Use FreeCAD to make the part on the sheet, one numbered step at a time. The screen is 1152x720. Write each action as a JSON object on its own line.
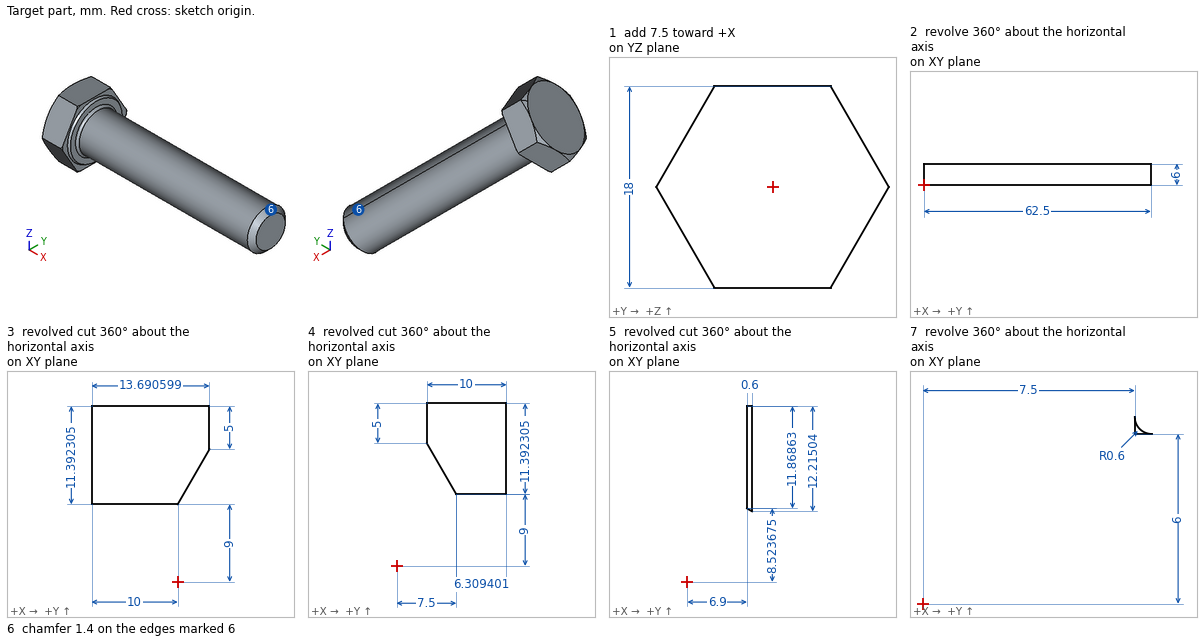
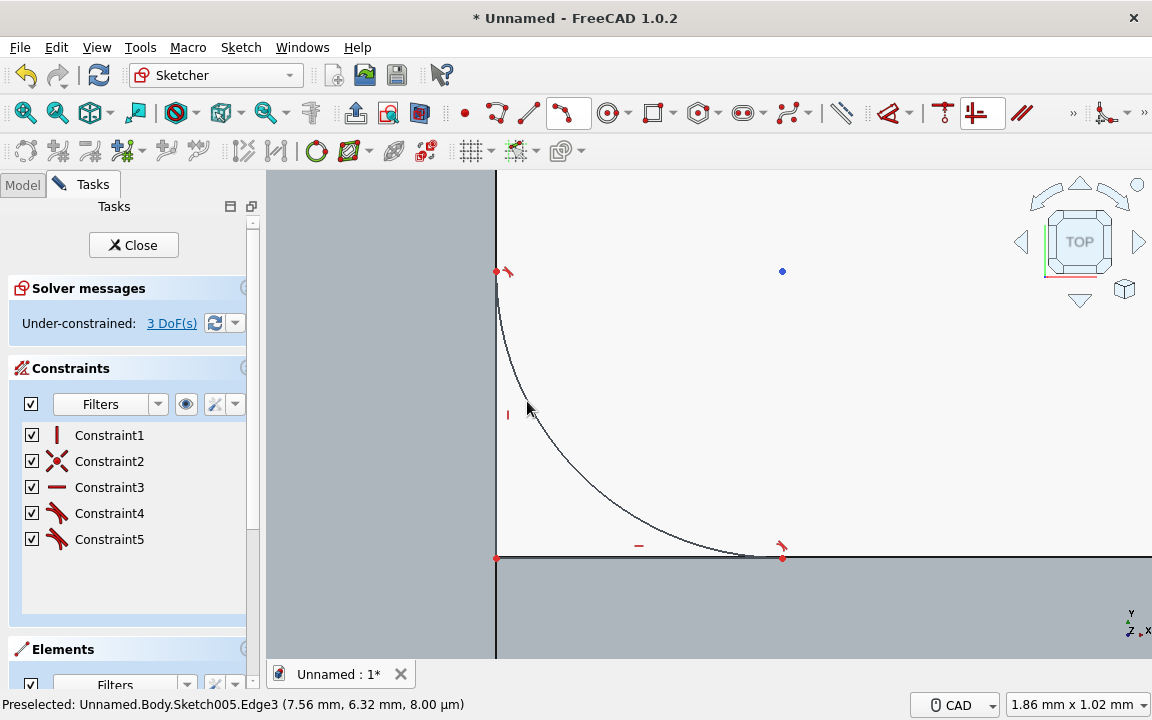
{"action": "key", "text": "d"}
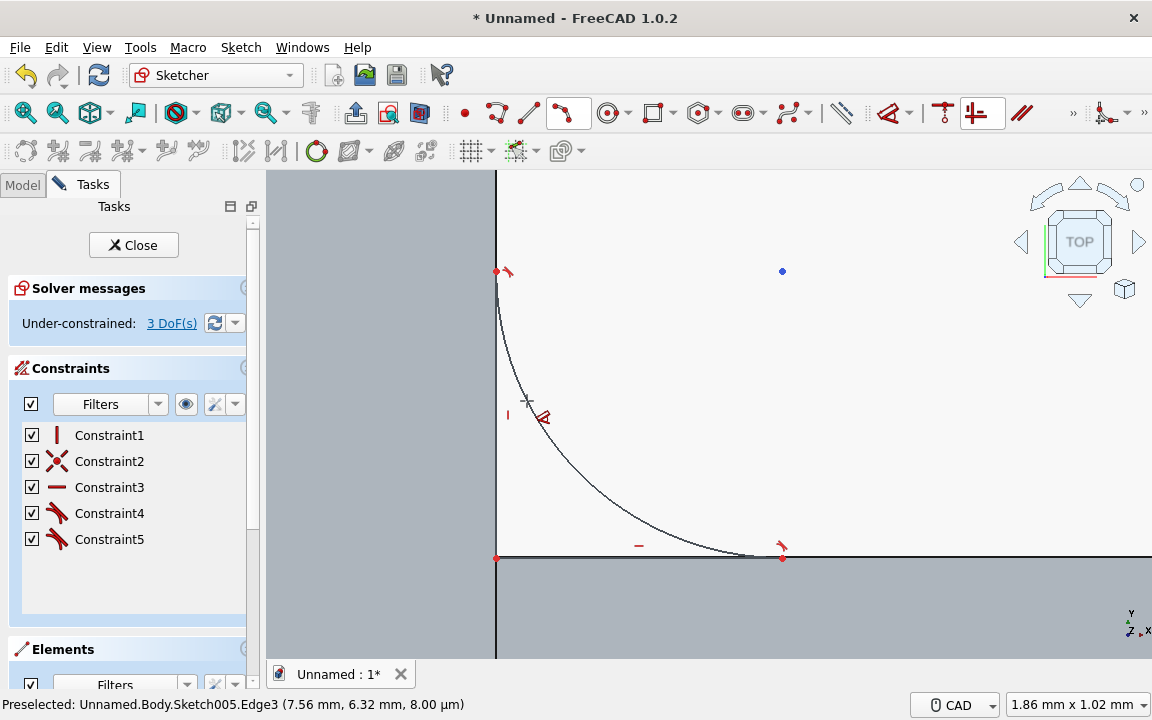
{"action": "left_click", "coordinate": [527, 401]}
{"action": "left_click", "coordinate": [464, 261]}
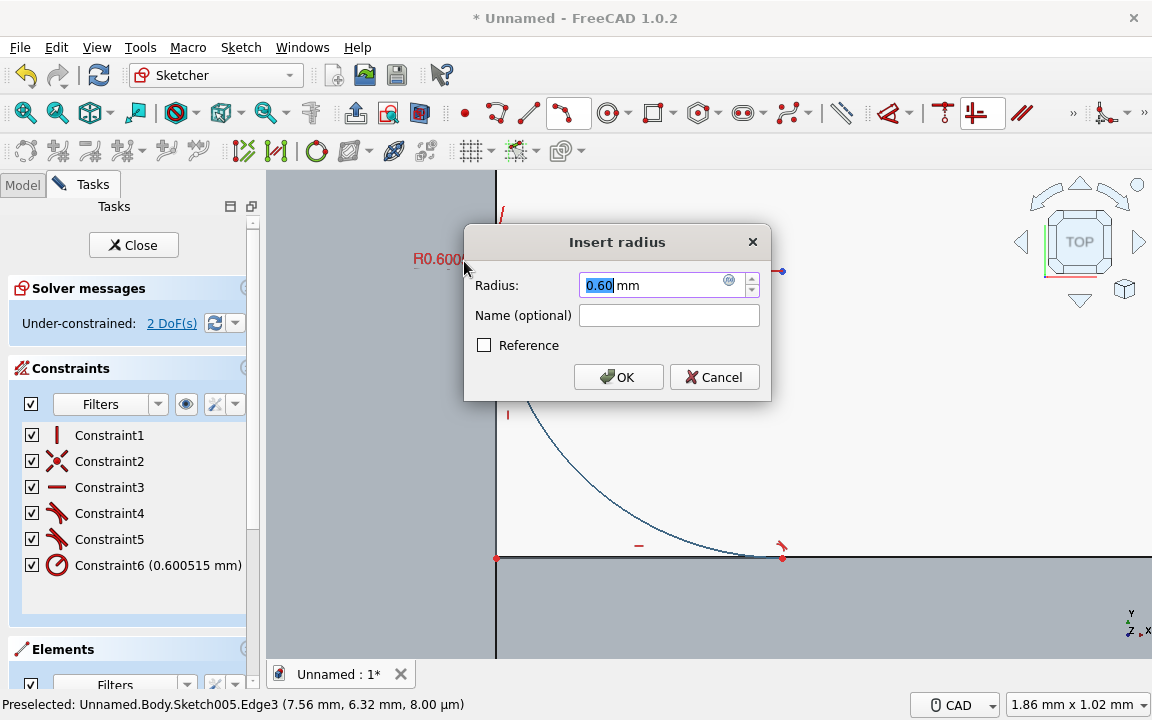
{"action": "type", "text": "0.6"}
{"action": "key", "text": "Return"}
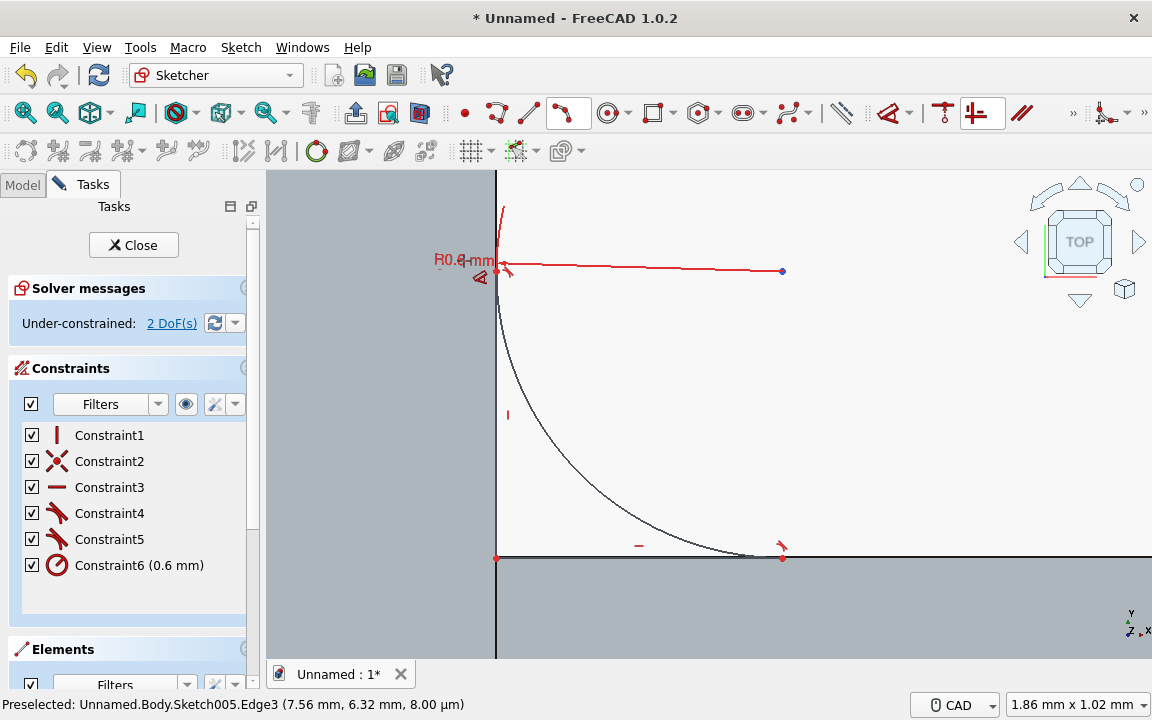
{"action": "left_click", "coordinate": [496, 558]}
{"action": "left_click", "coordinate": [530, 595]}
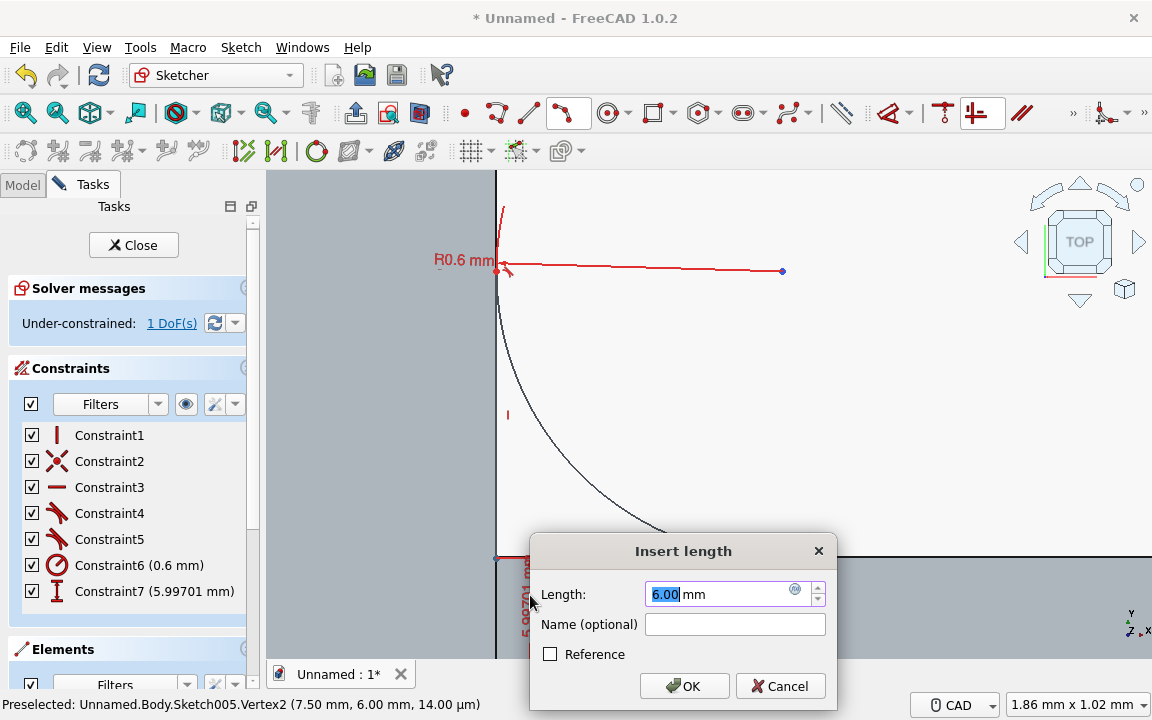
{"action": "type", "text": "6"}
{"action": "key", "text": "Return"}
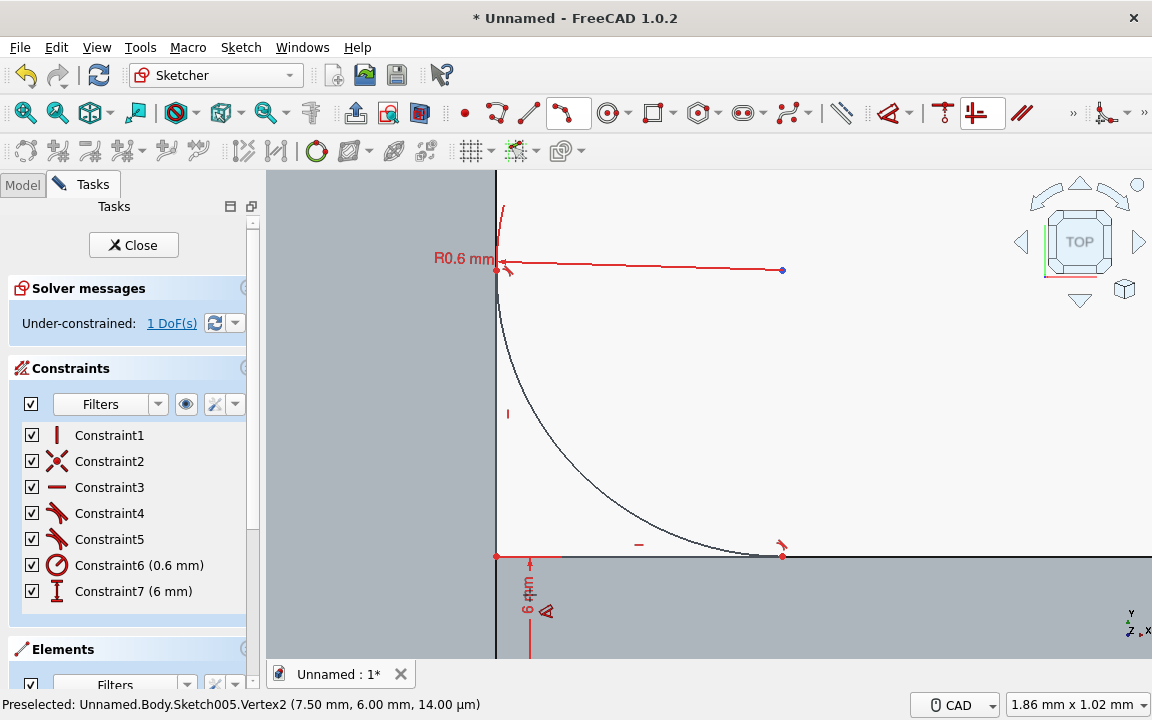
{"action": "left_click", "coordinate": [496, 270]}
{"action": "left_click", "coordinate": [395, 236]}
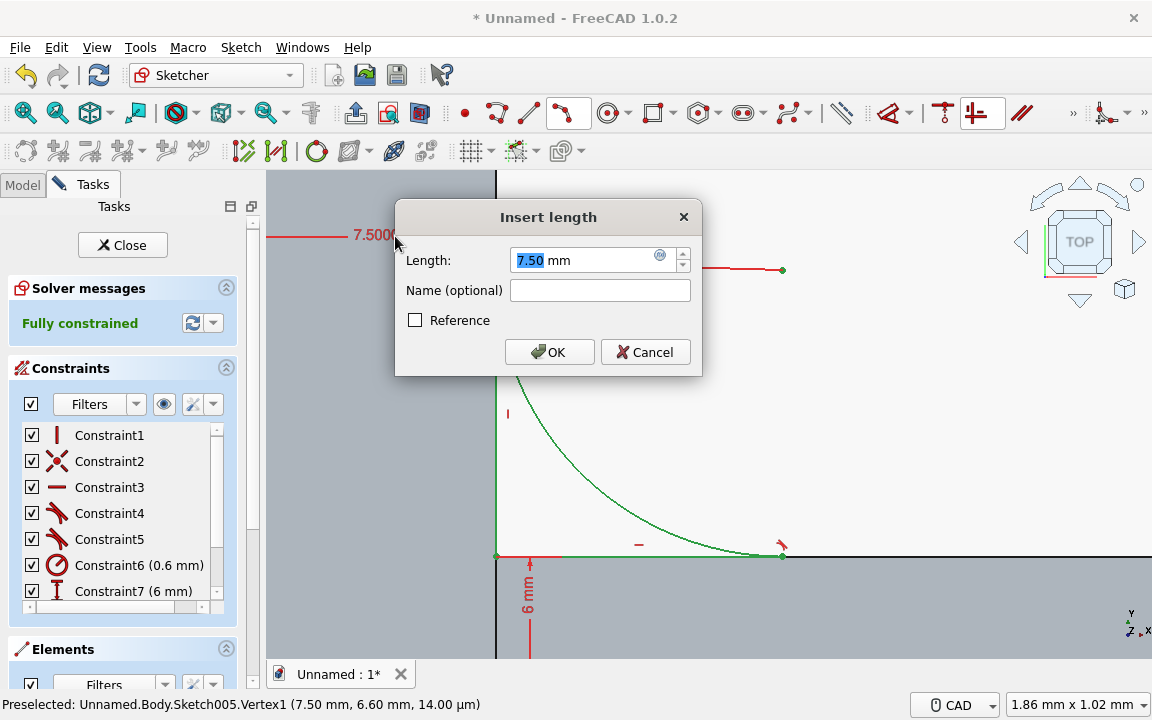
{"action": "type", "text": "7.5"}
{"action": "key", "text": "Return"}
{"action": "key", "text": "Escape"}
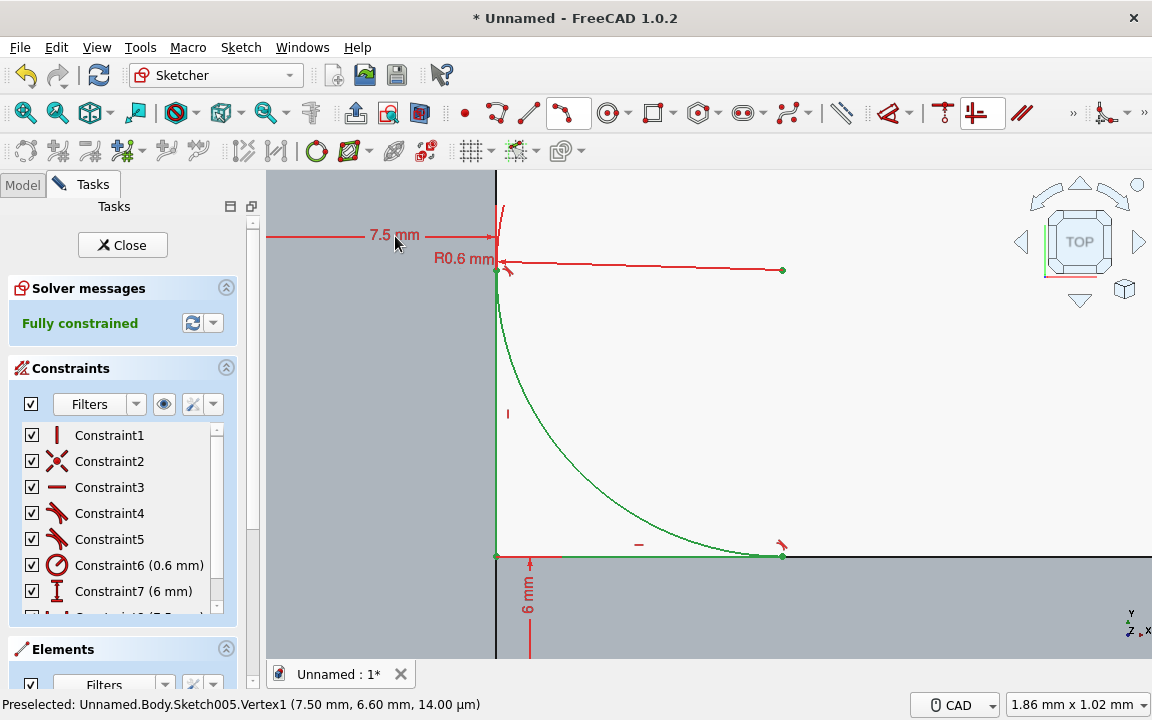
{"action": "left_click", "coordinate": [123, 245]}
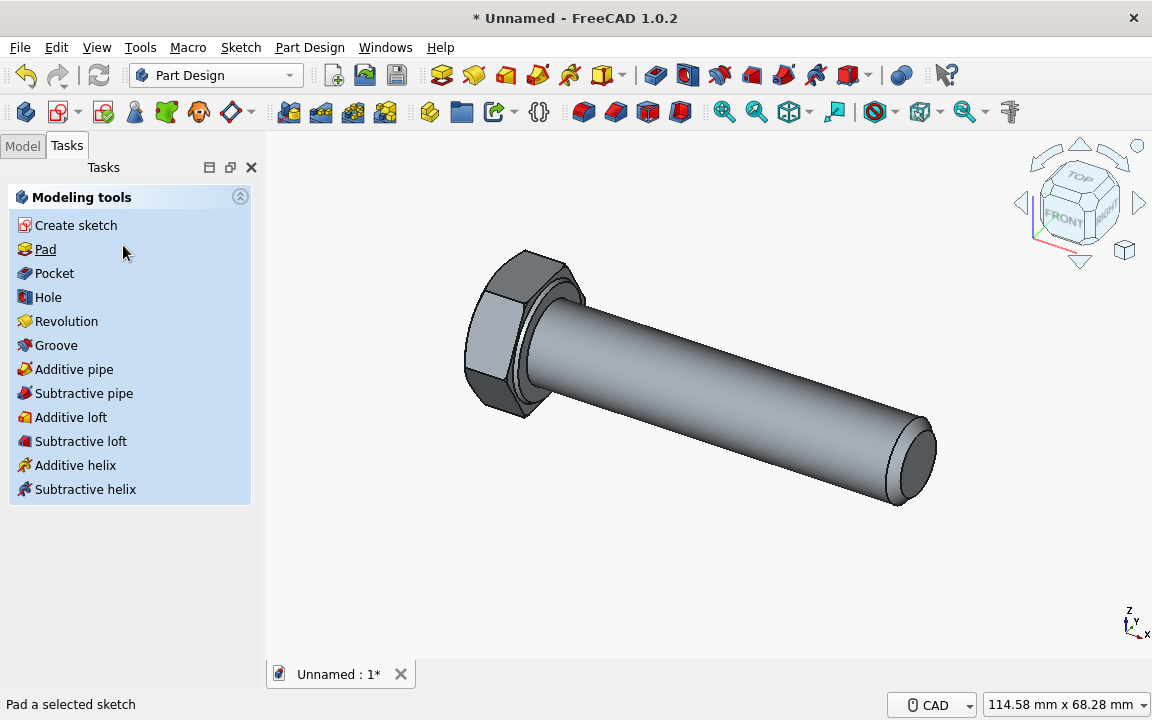
{"action": "left_click", "coordinate": [474, 76]}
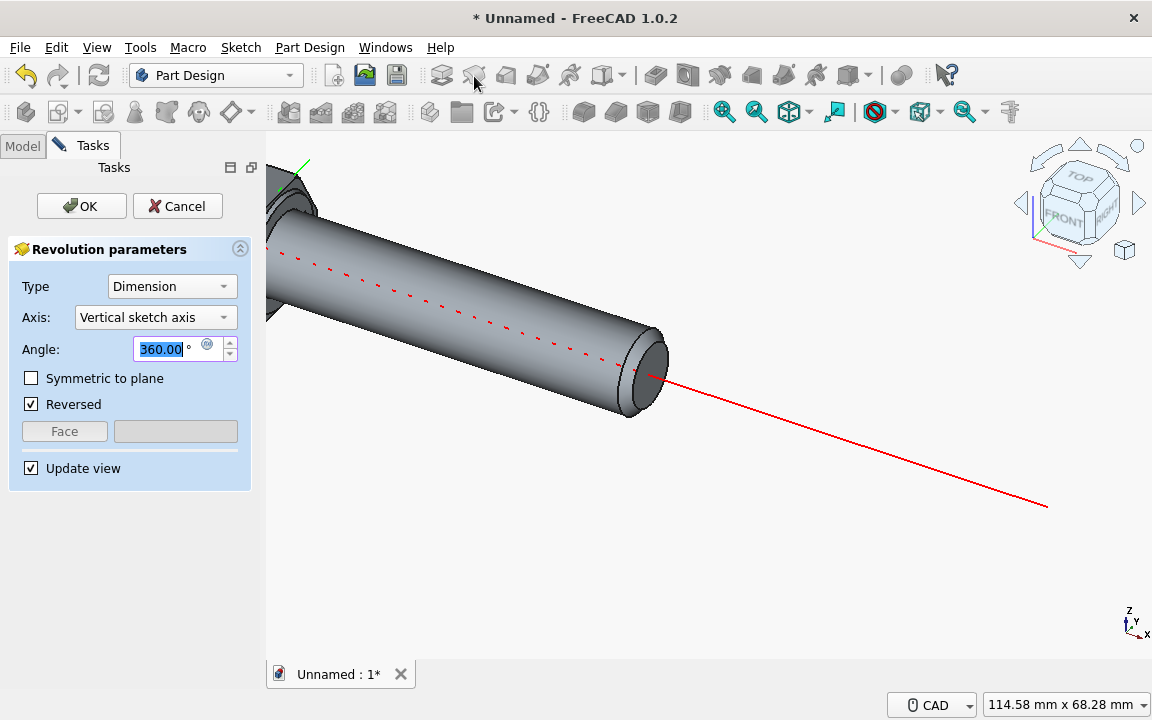
{"action": "left_click", "coordinate": [156, 318]}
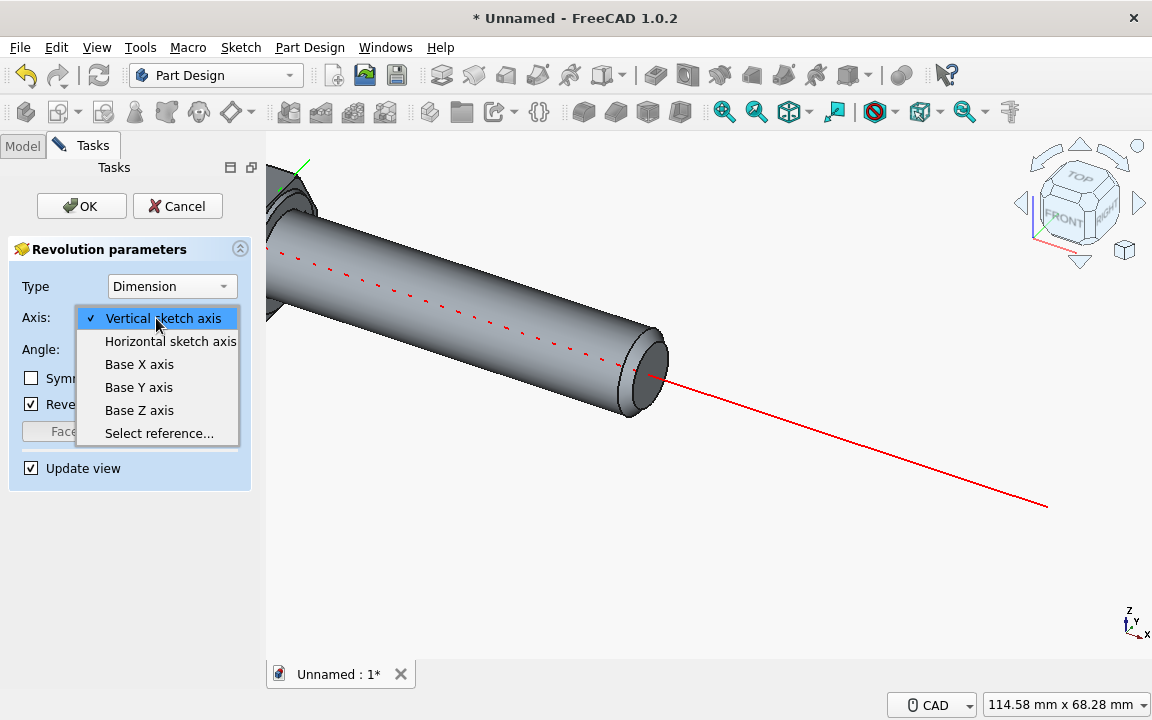
{"action": "left_click", "coordinate": [156, 342]}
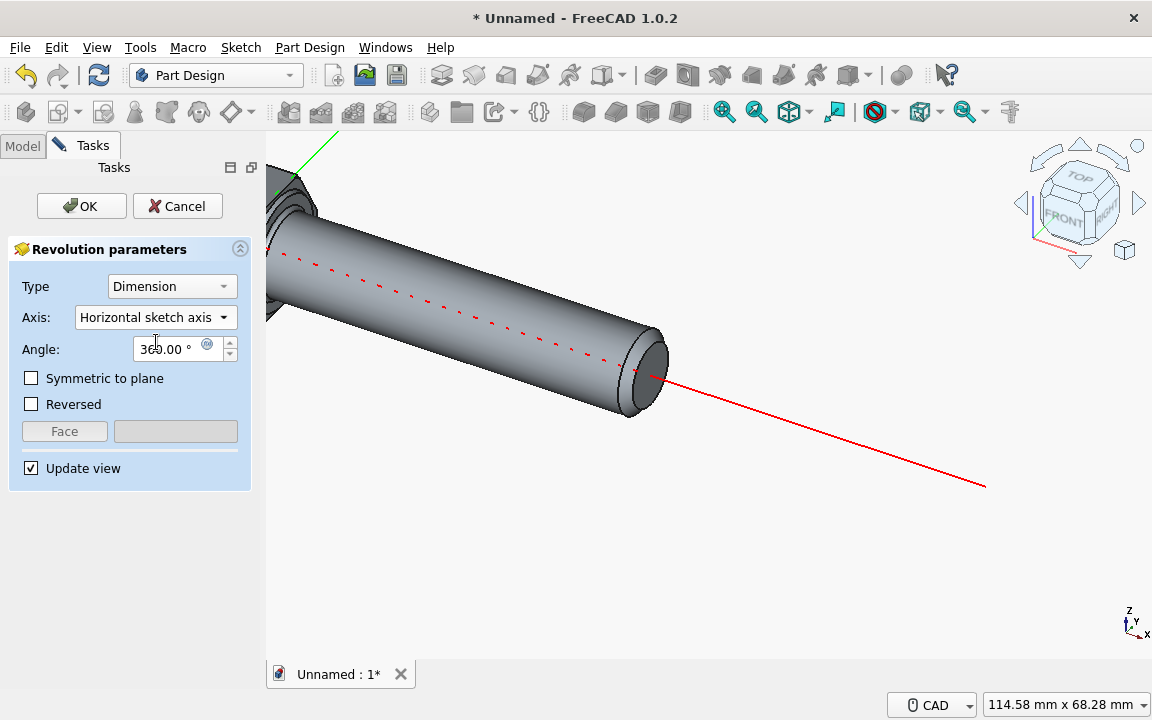
{"action": "left_click", "coordinate": [82, 206]}